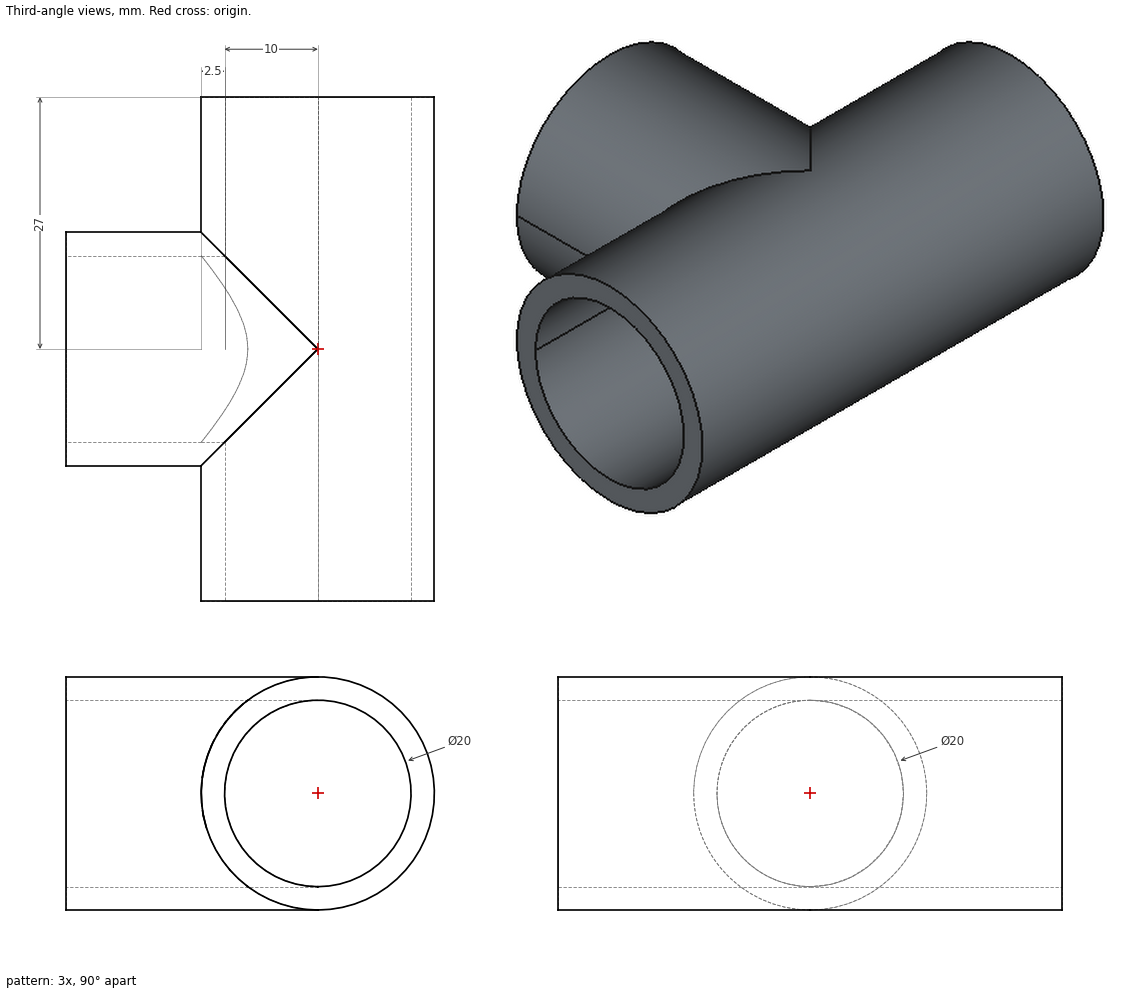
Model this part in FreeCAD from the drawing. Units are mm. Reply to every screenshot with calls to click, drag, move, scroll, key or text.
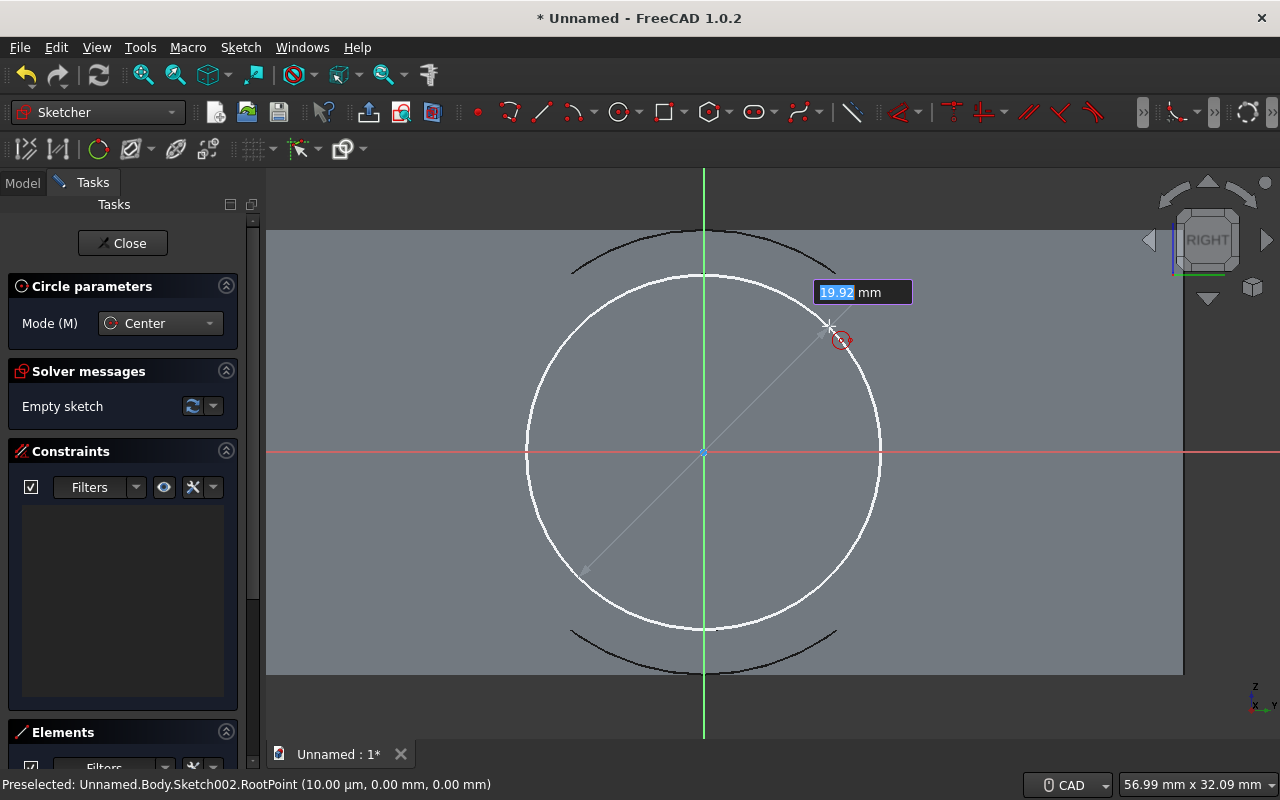
text(20)
key(Return)
key(Escape)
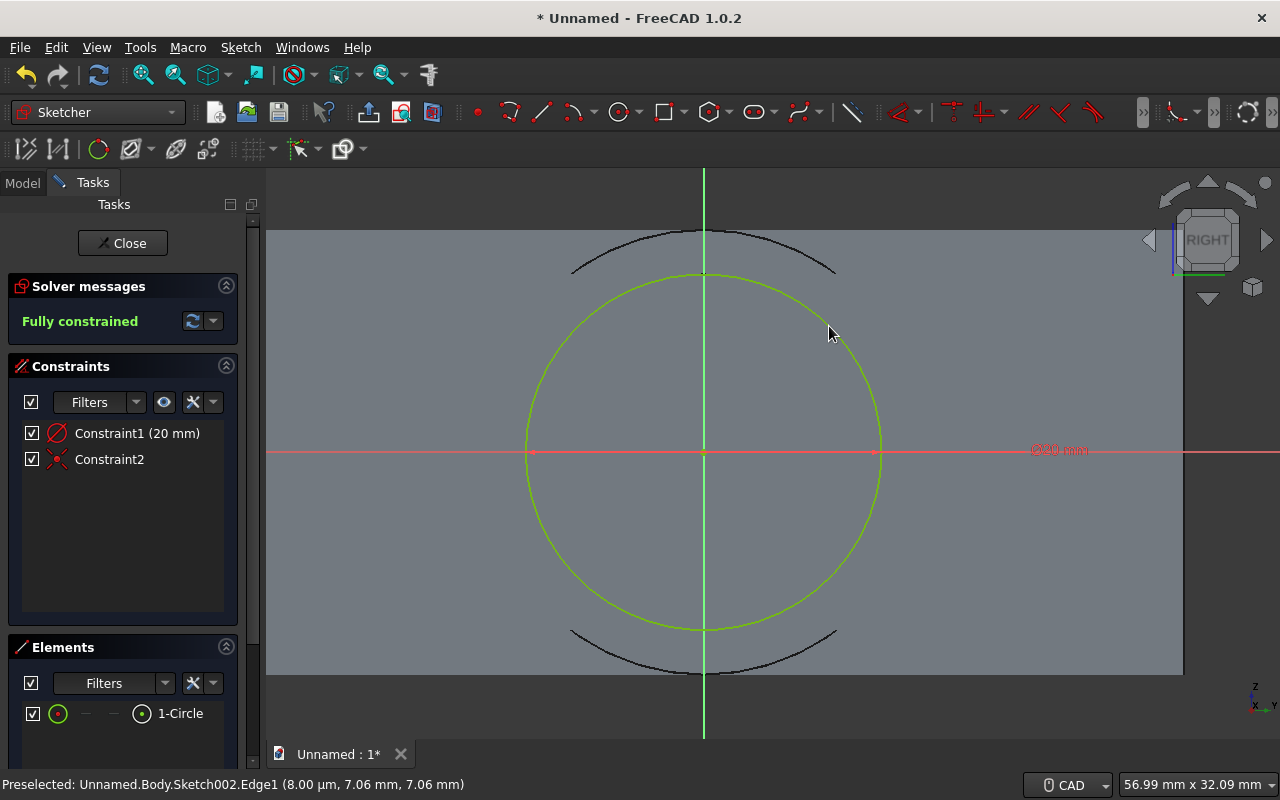
click(123, 243)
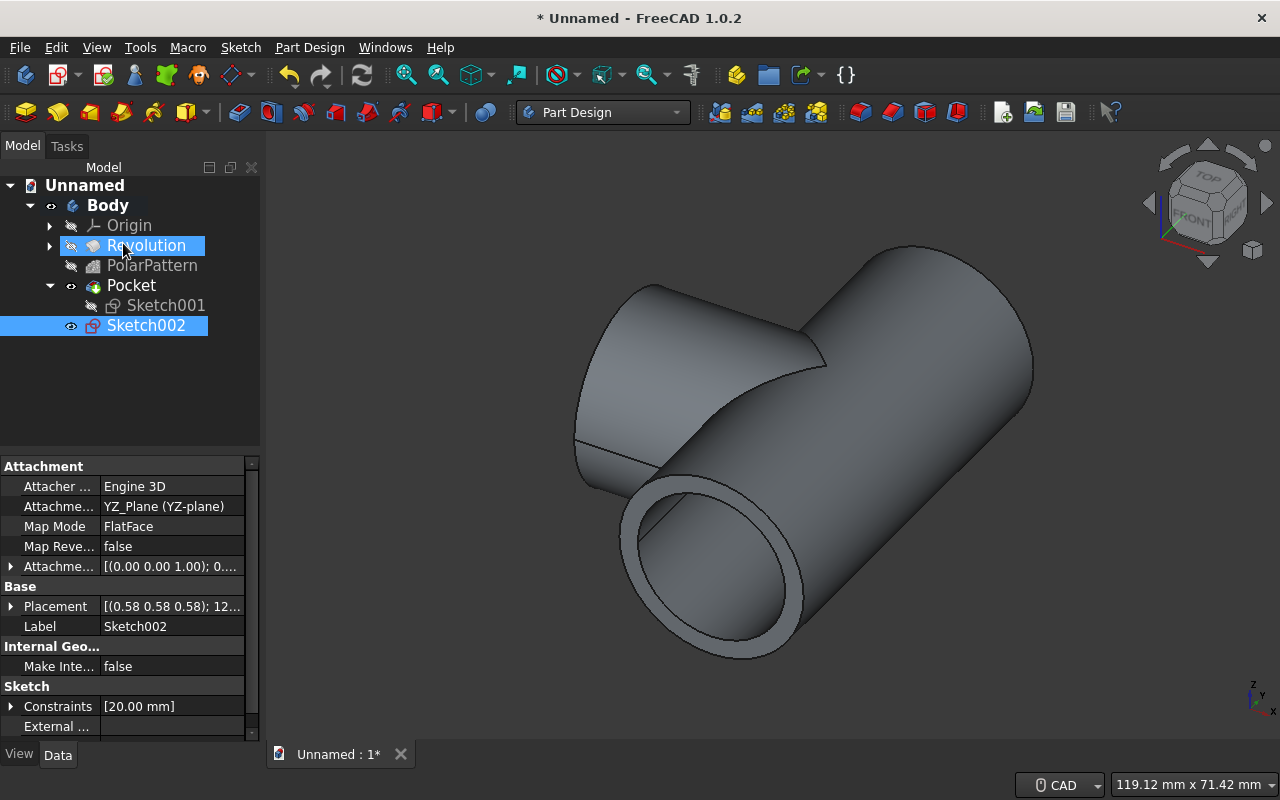
click(240, 112)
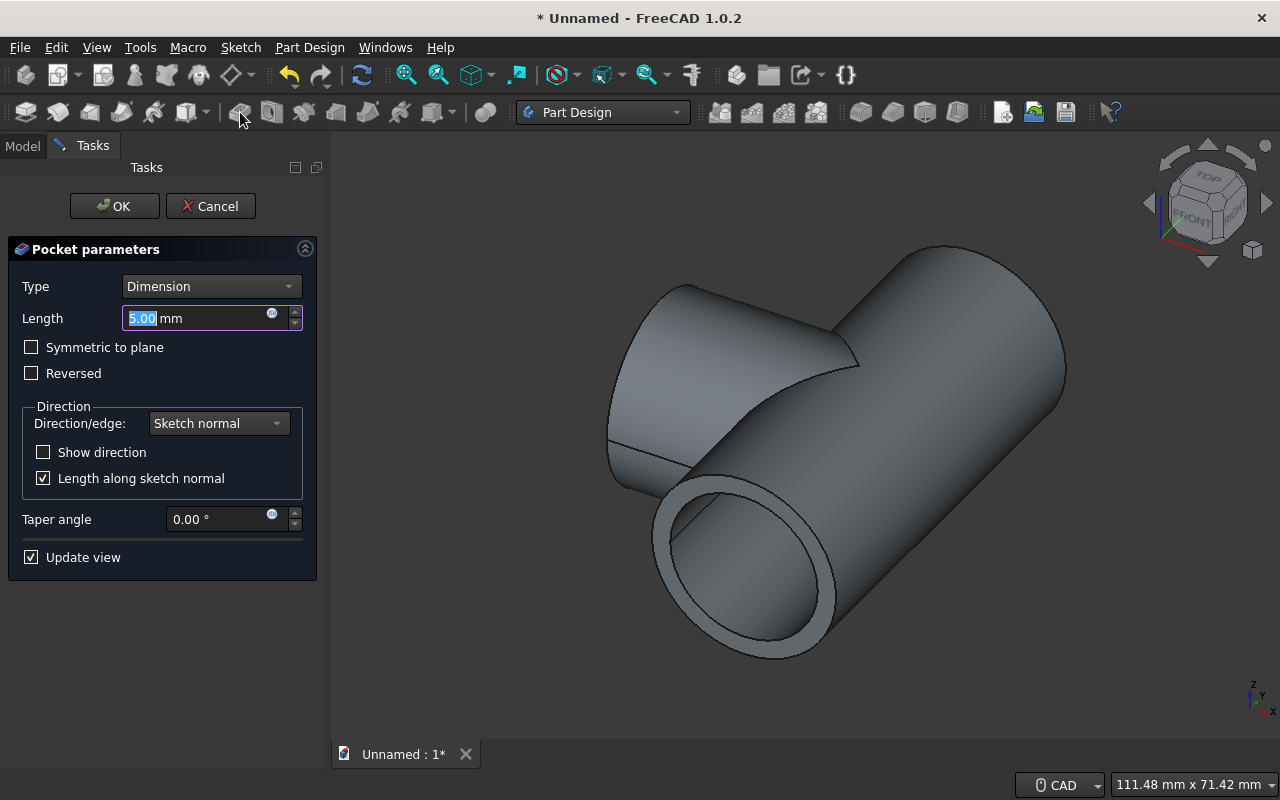
click(212, 286)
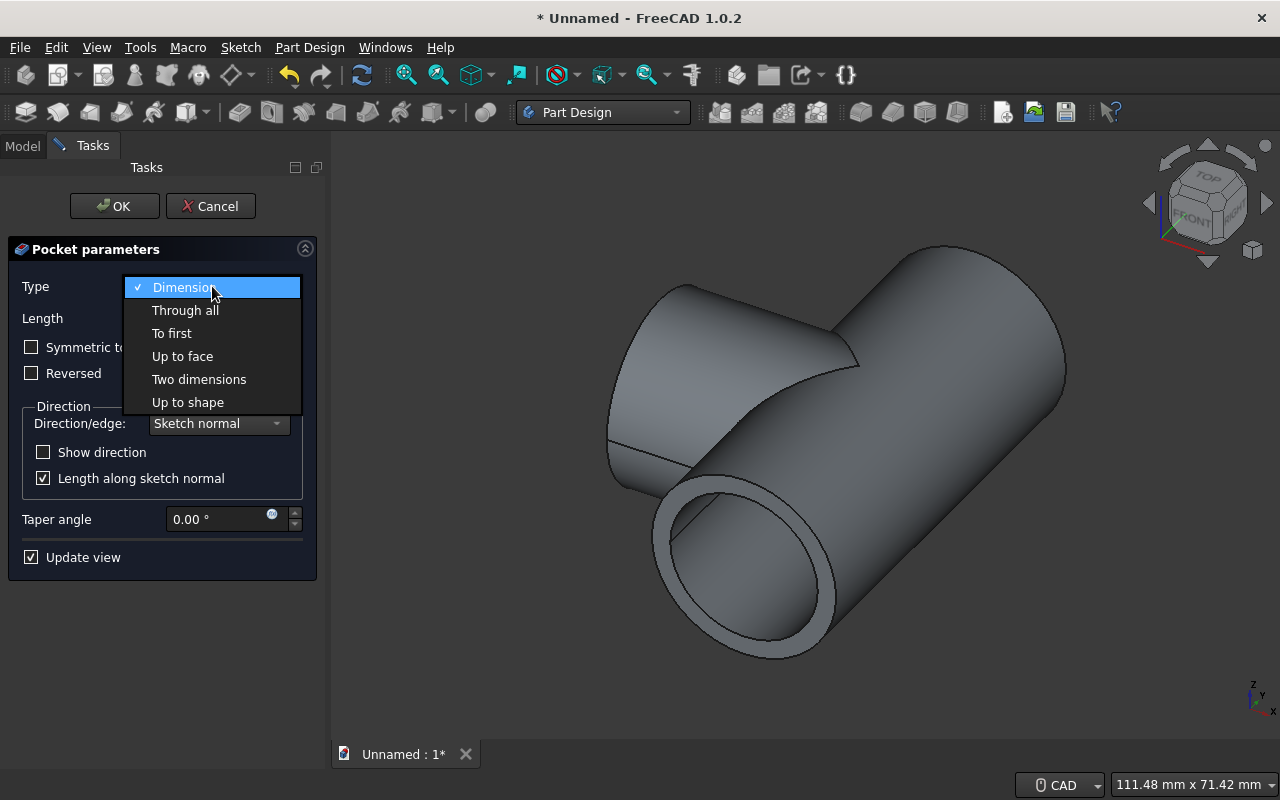
click(212, 310)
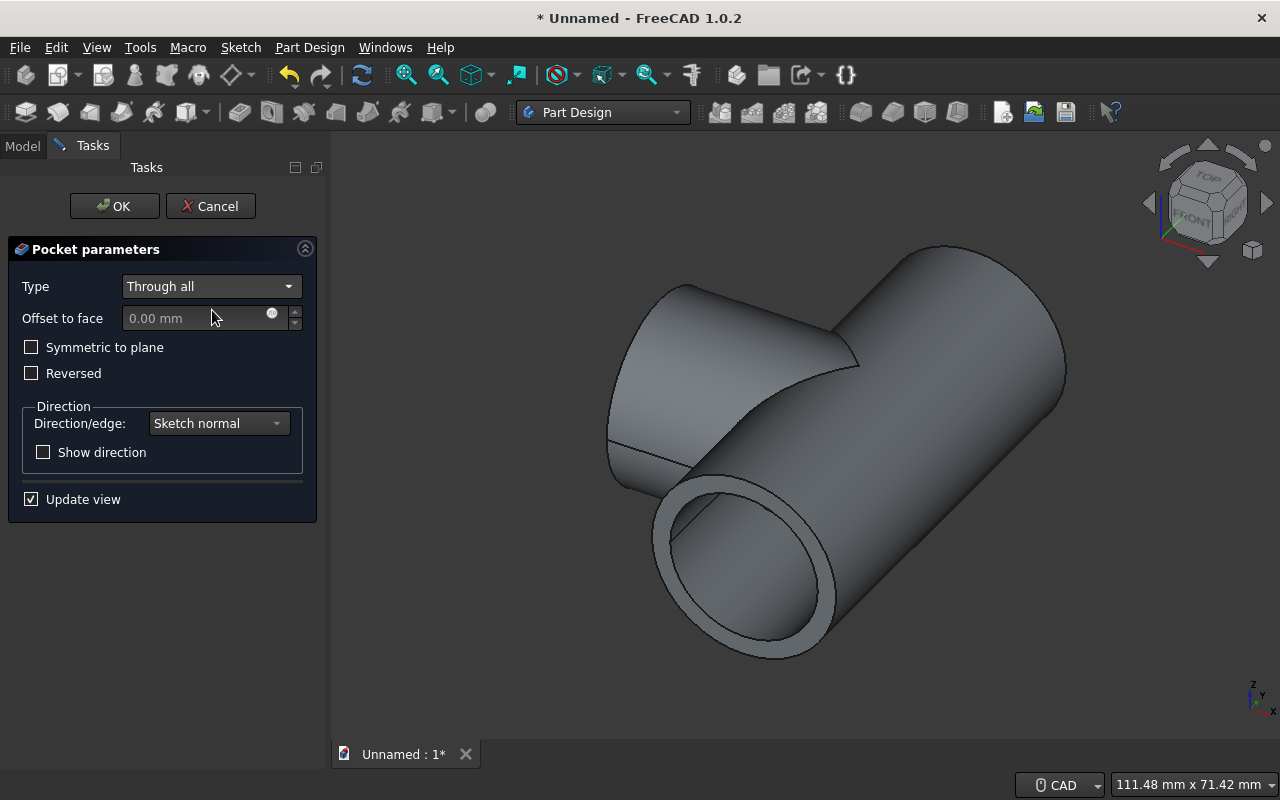
click(115, 206)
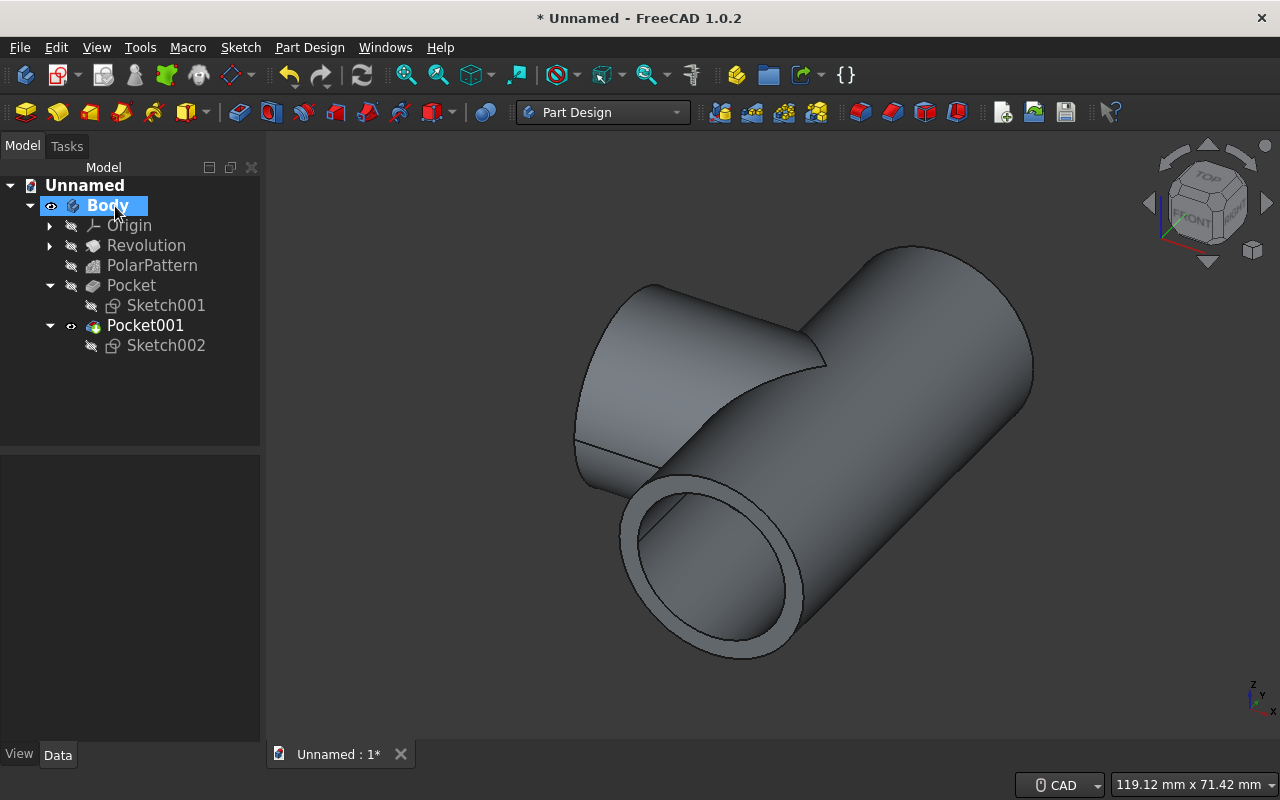
key(0)